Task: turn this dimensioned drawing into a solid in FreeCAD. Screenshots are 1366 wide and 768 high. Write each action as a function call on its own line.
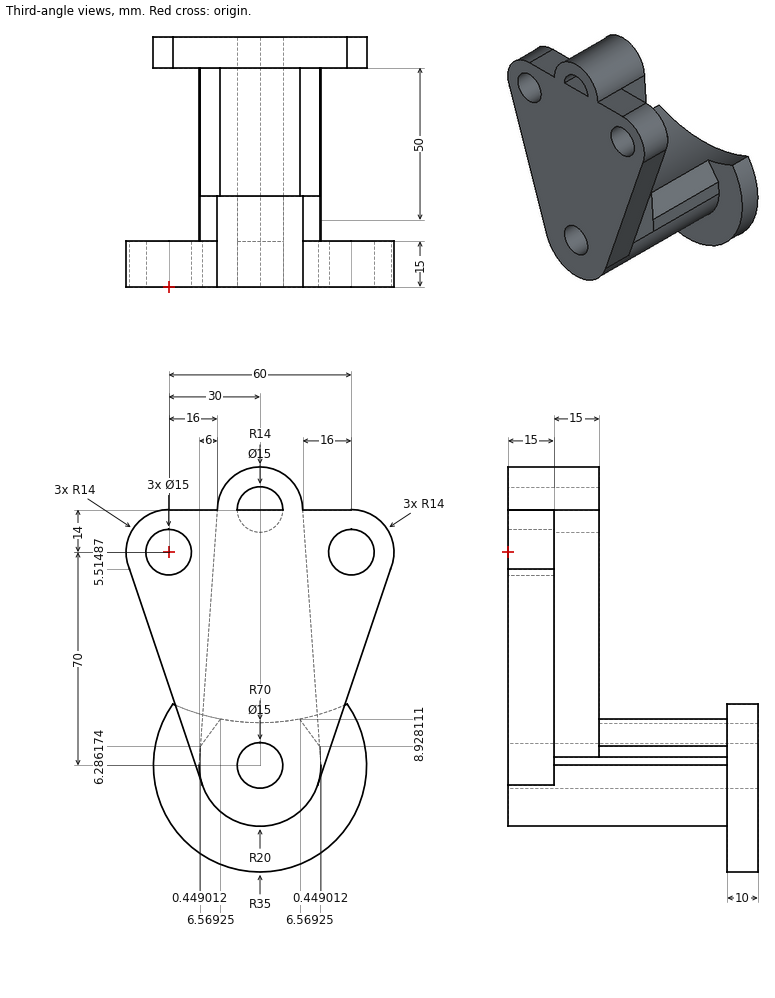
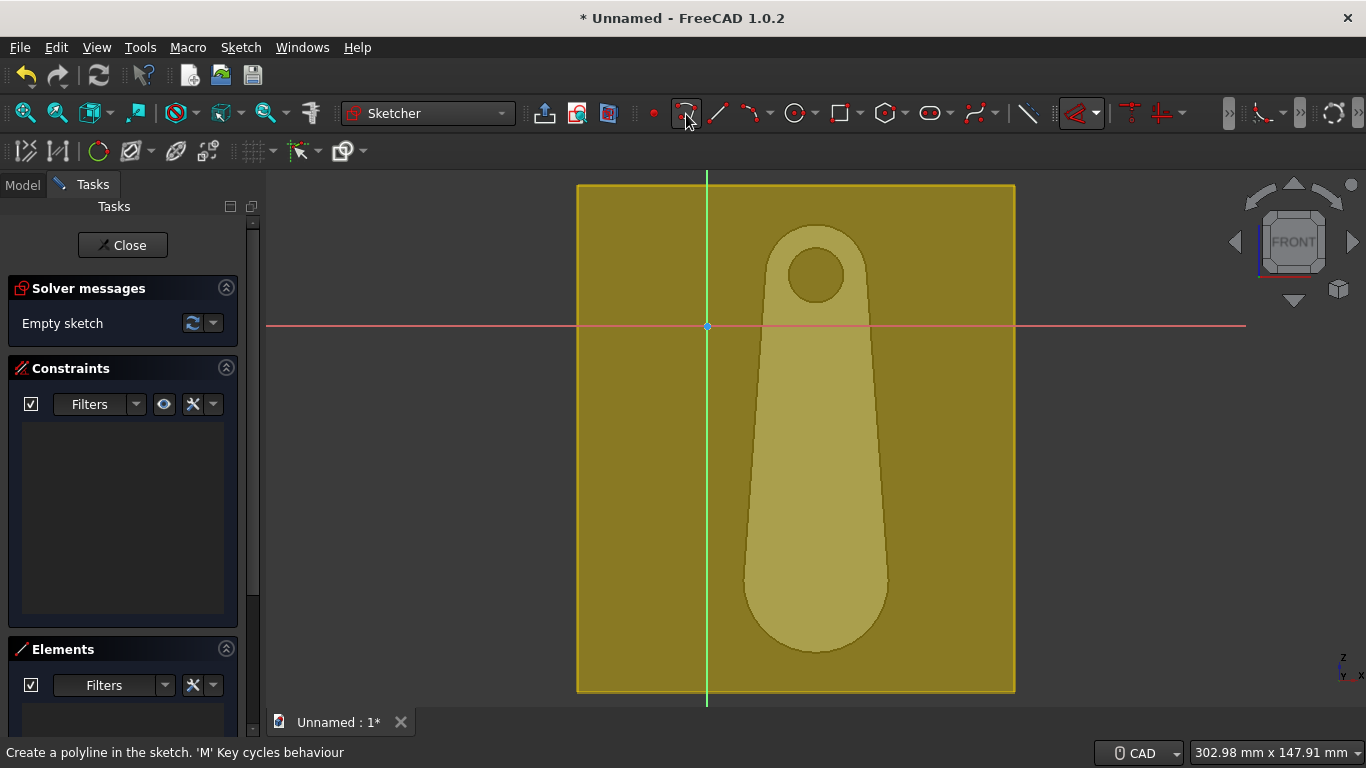
click(863, 525)
click(887, 557)
click(890, 580)
right_click(890, 580)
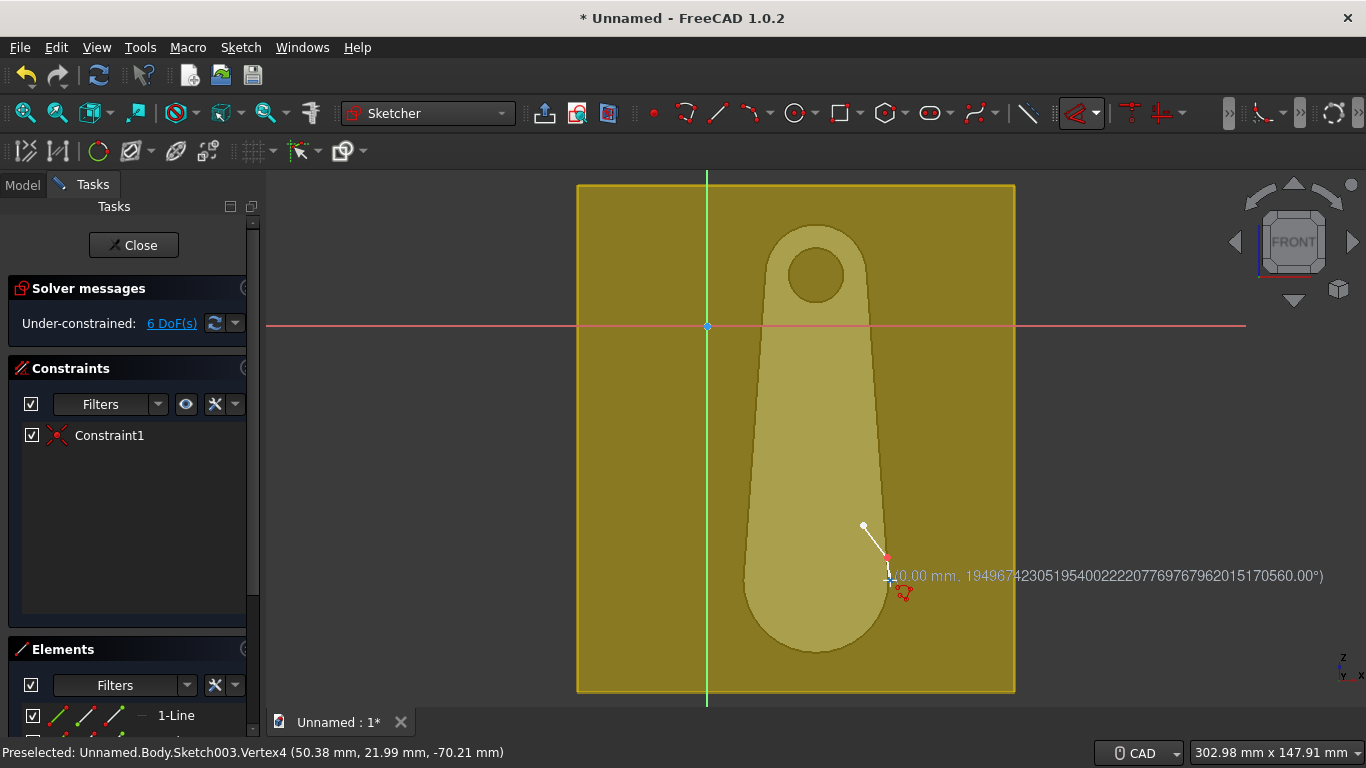
click(743, 580)
click(746, 557)
click(769, 525)
right_click(769, 525)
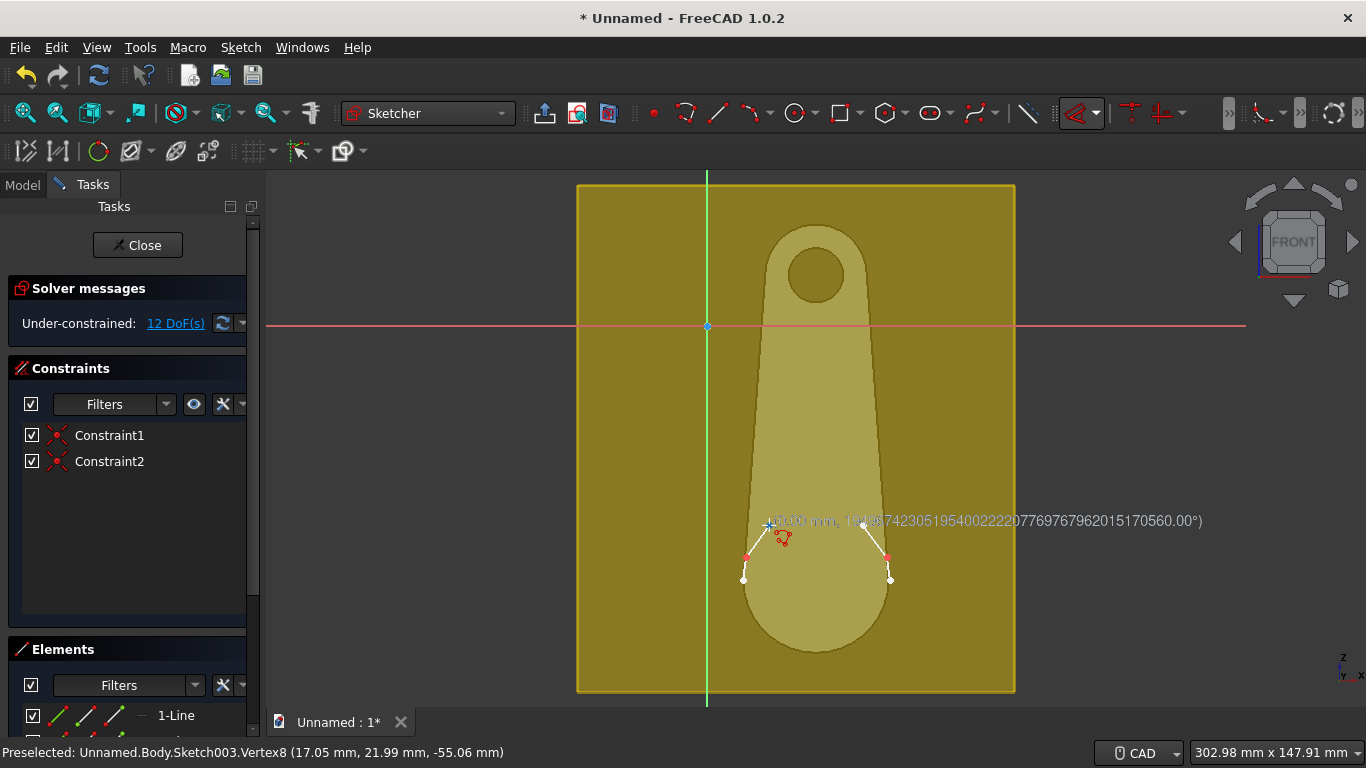
click(750, 114)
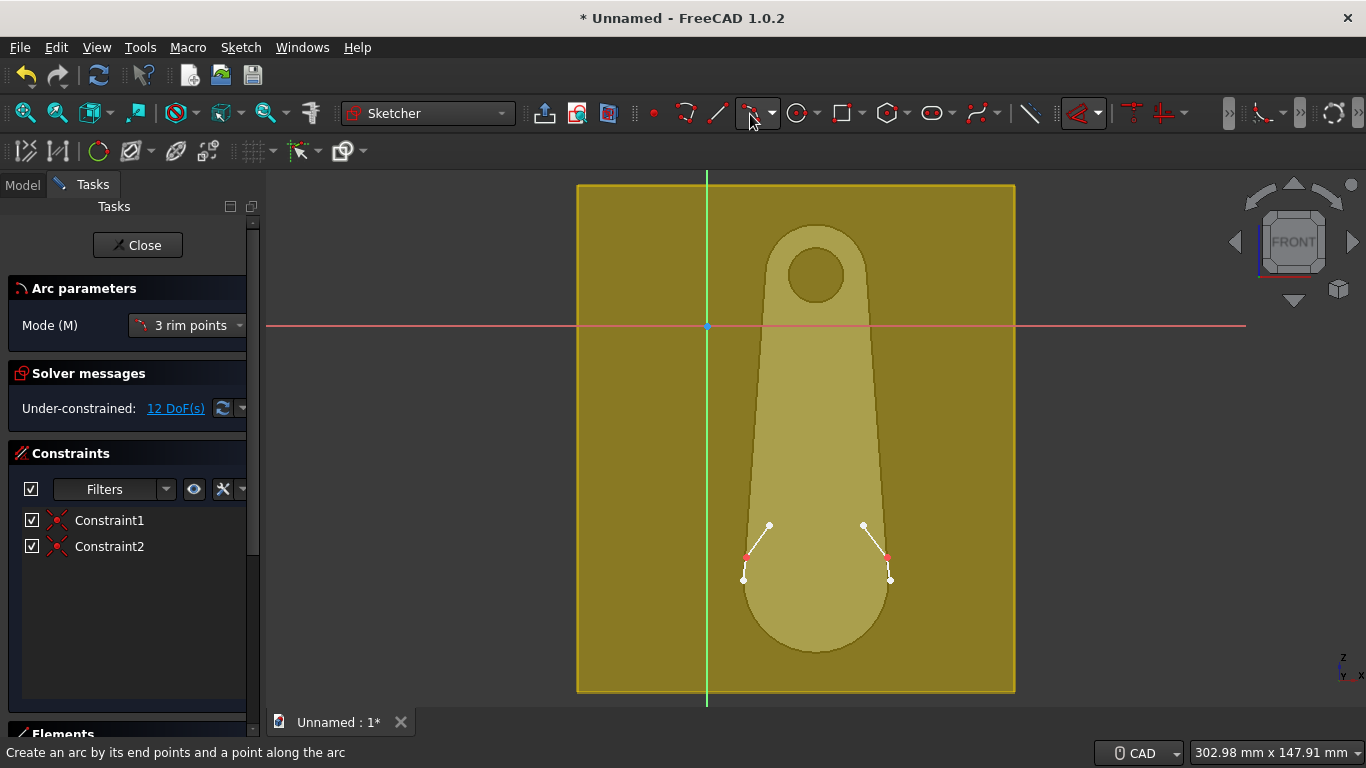
scroll(889, 580, up, 2)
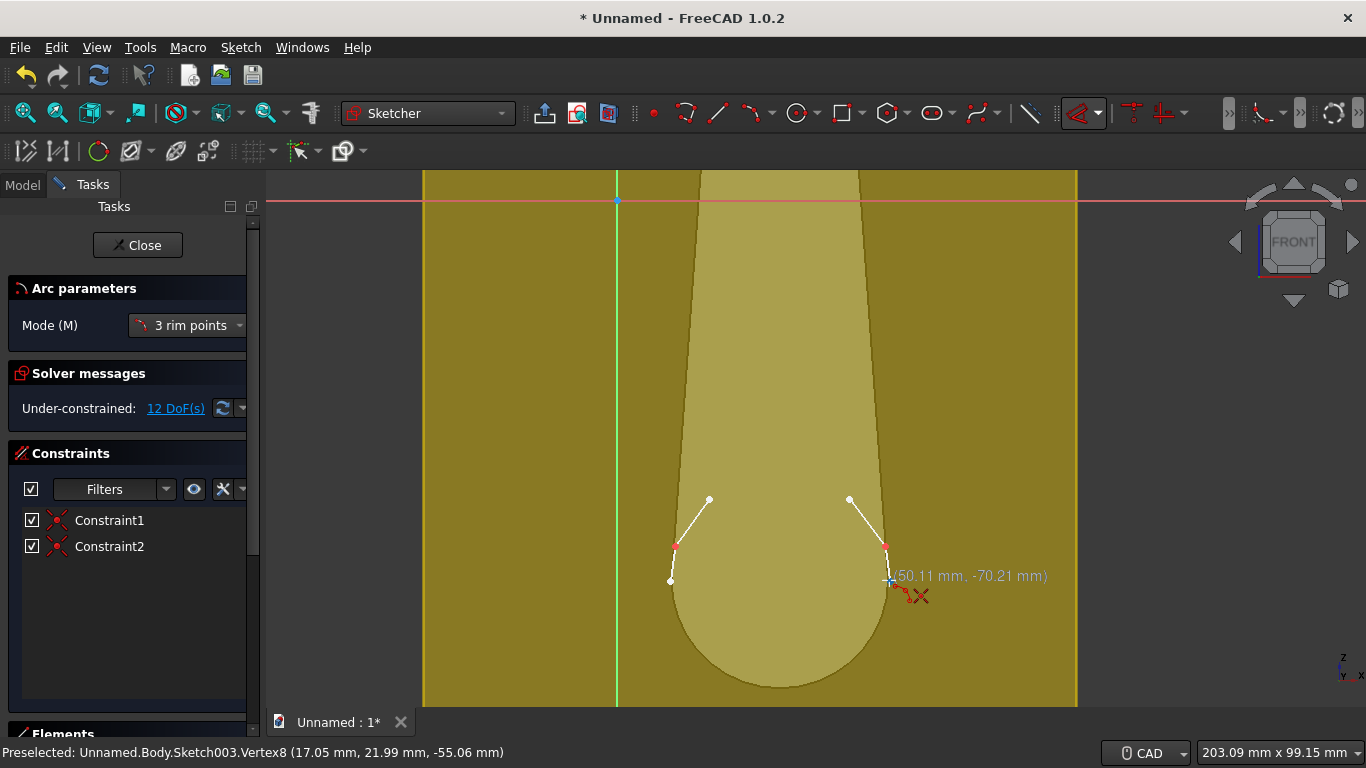
click(890, 581)
click(671, 581)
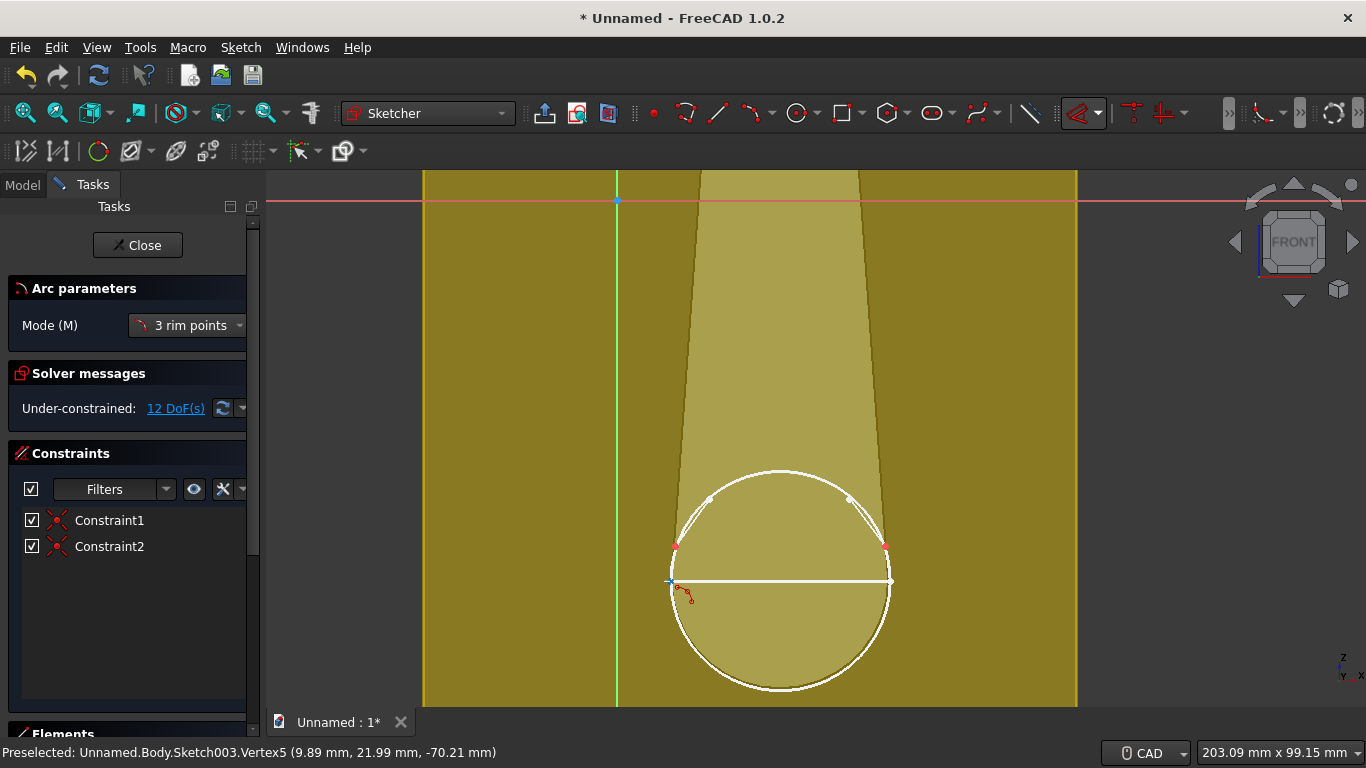
scroll(737, 426, down, 2)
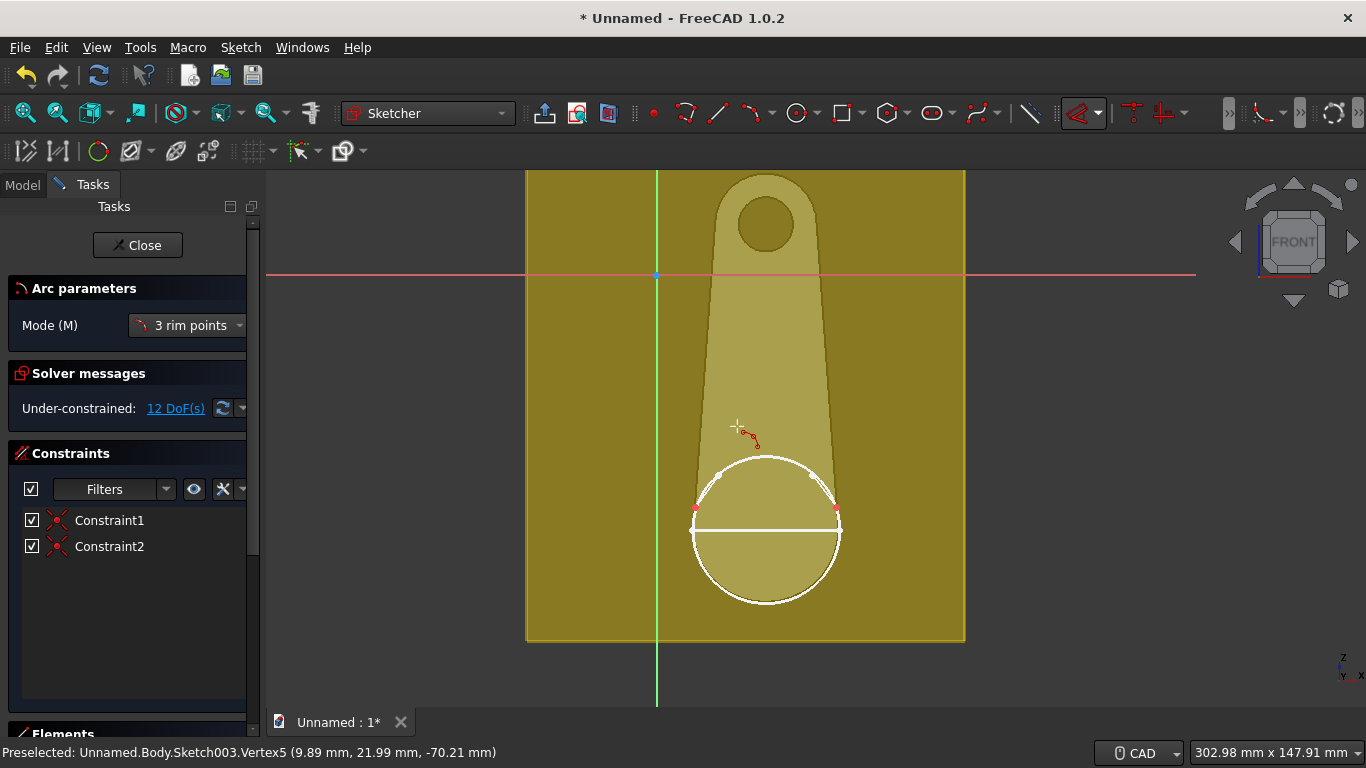
click(766, 602)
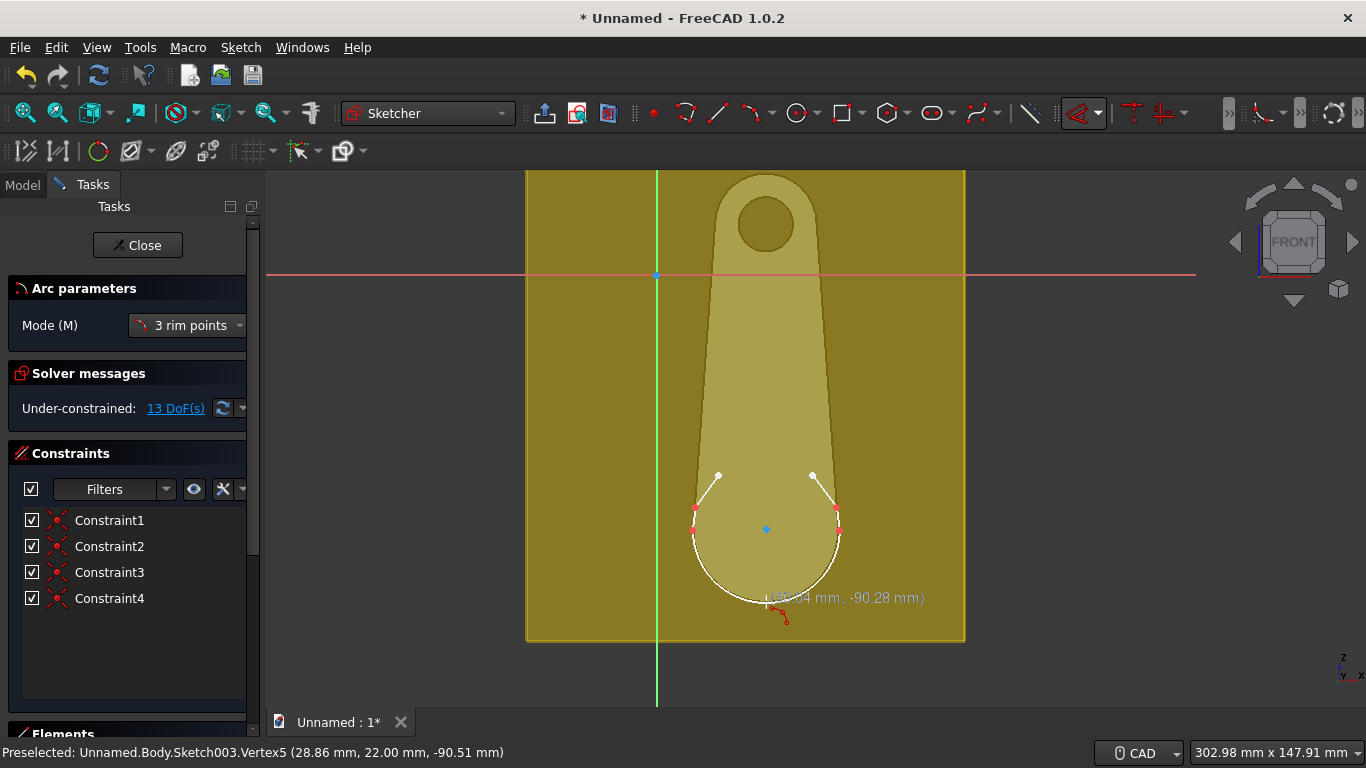
click(719, 475)
click(813, 475)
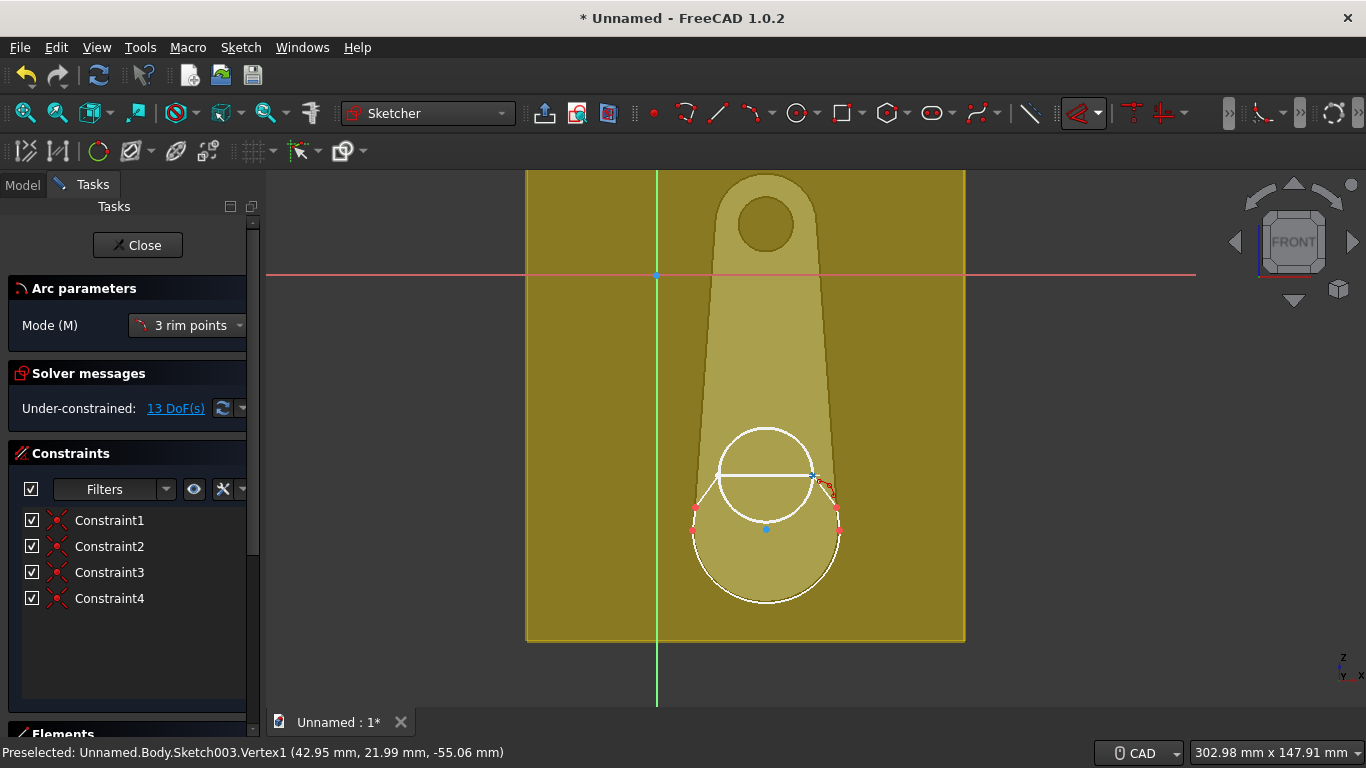
scroll(766, 479, up, 7)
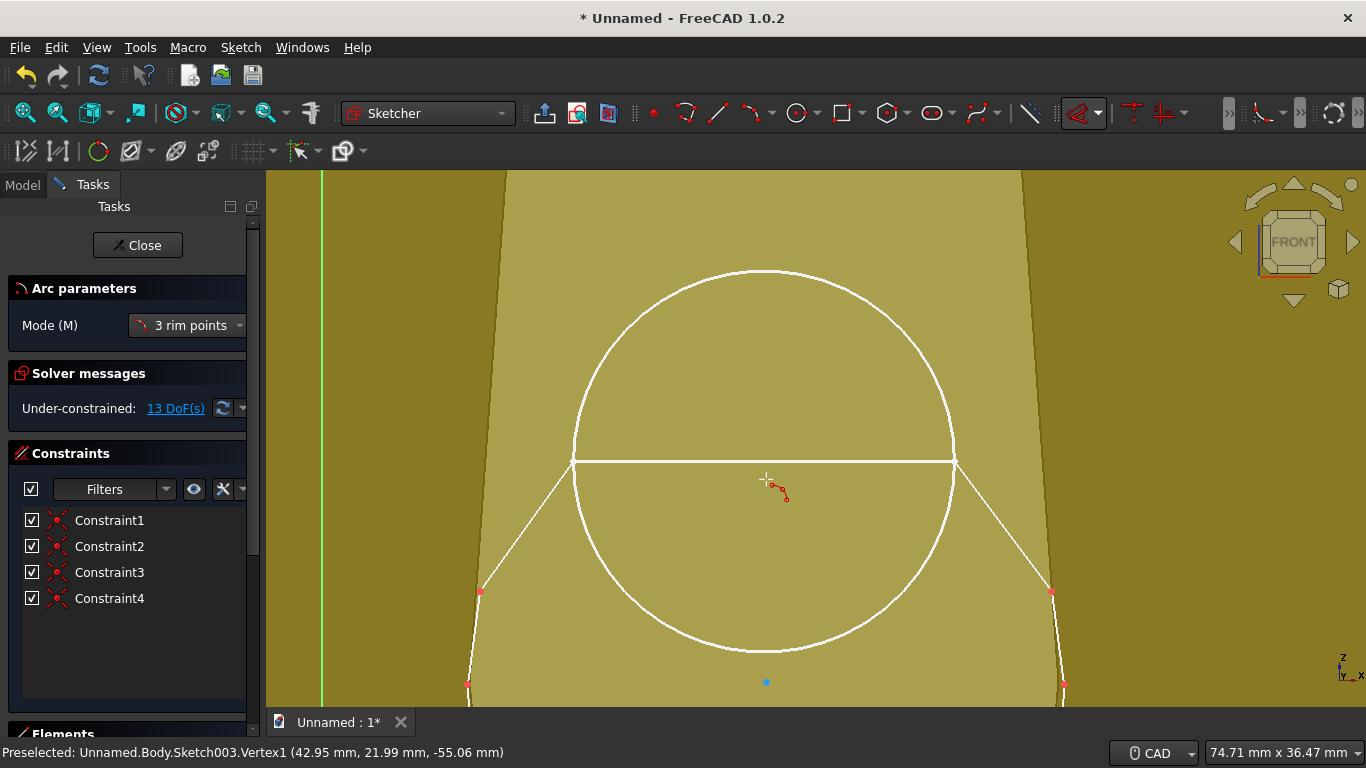
click(764, 475)